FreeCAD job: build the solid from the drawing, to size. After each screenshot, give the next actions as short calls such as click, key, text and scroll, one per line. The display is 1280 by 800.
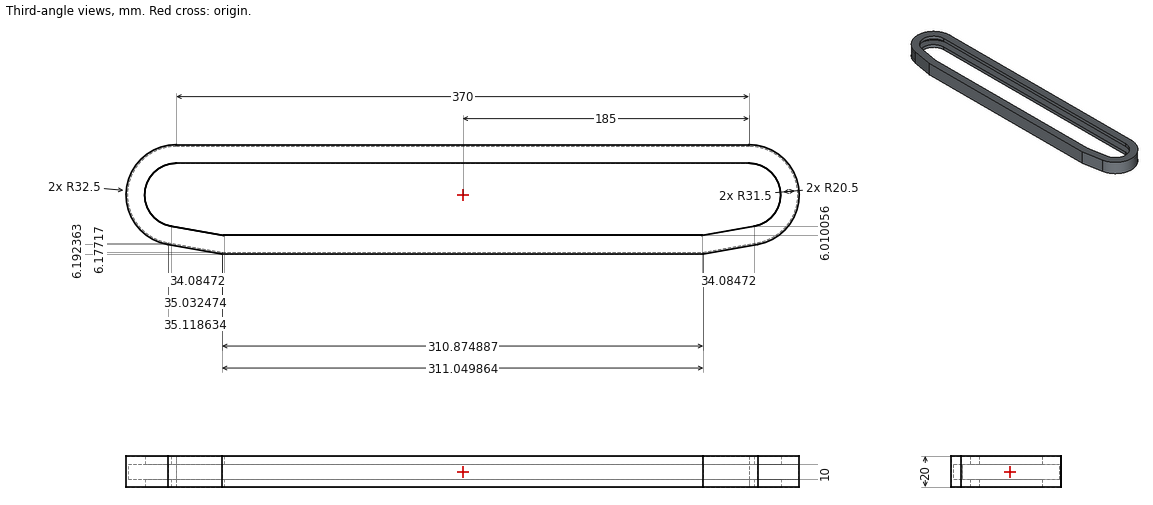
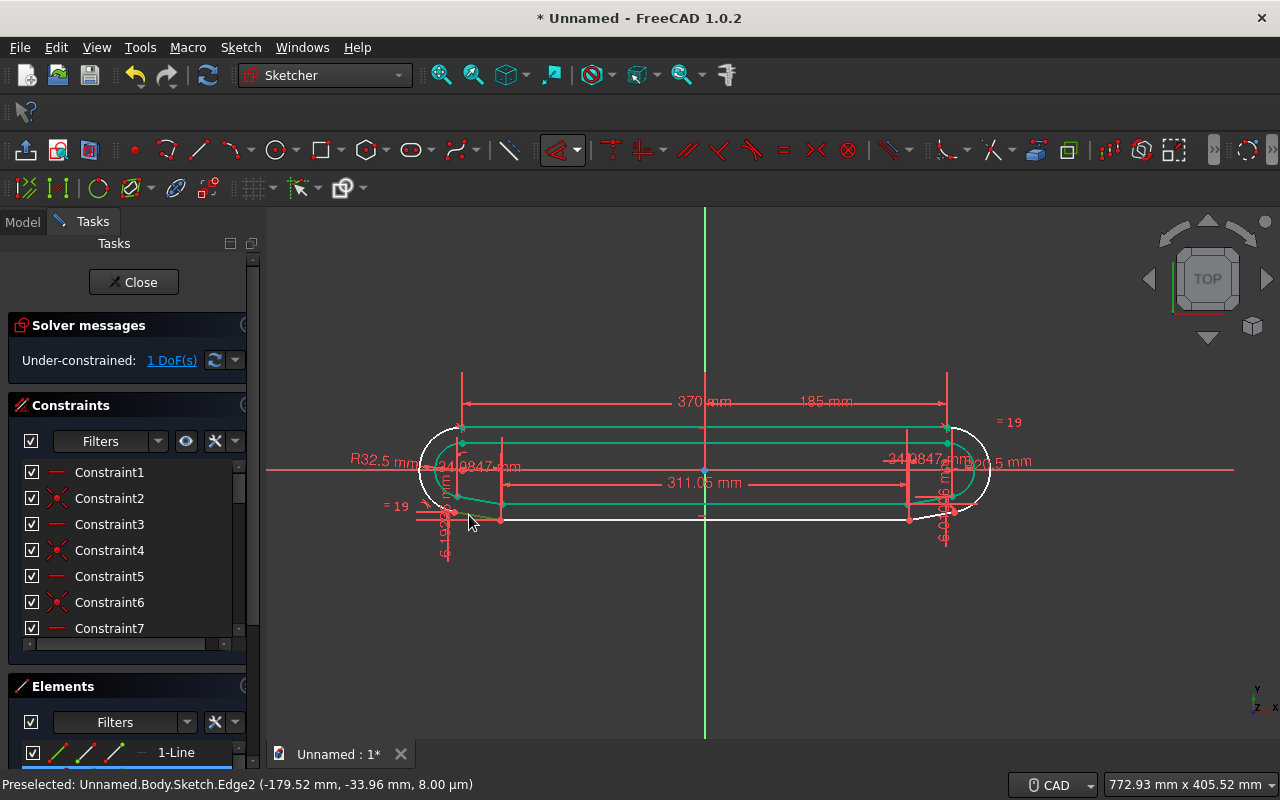
key(l)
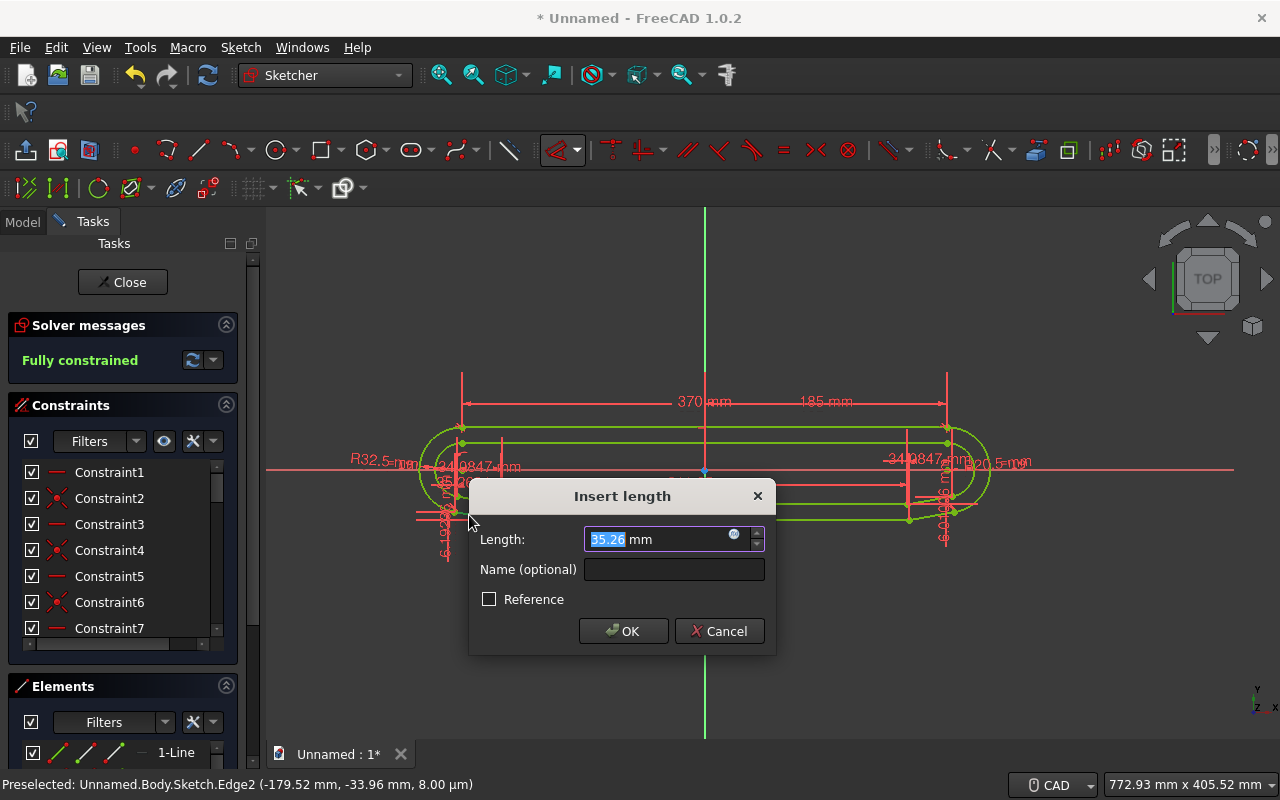
text(35.118634)
key(Return)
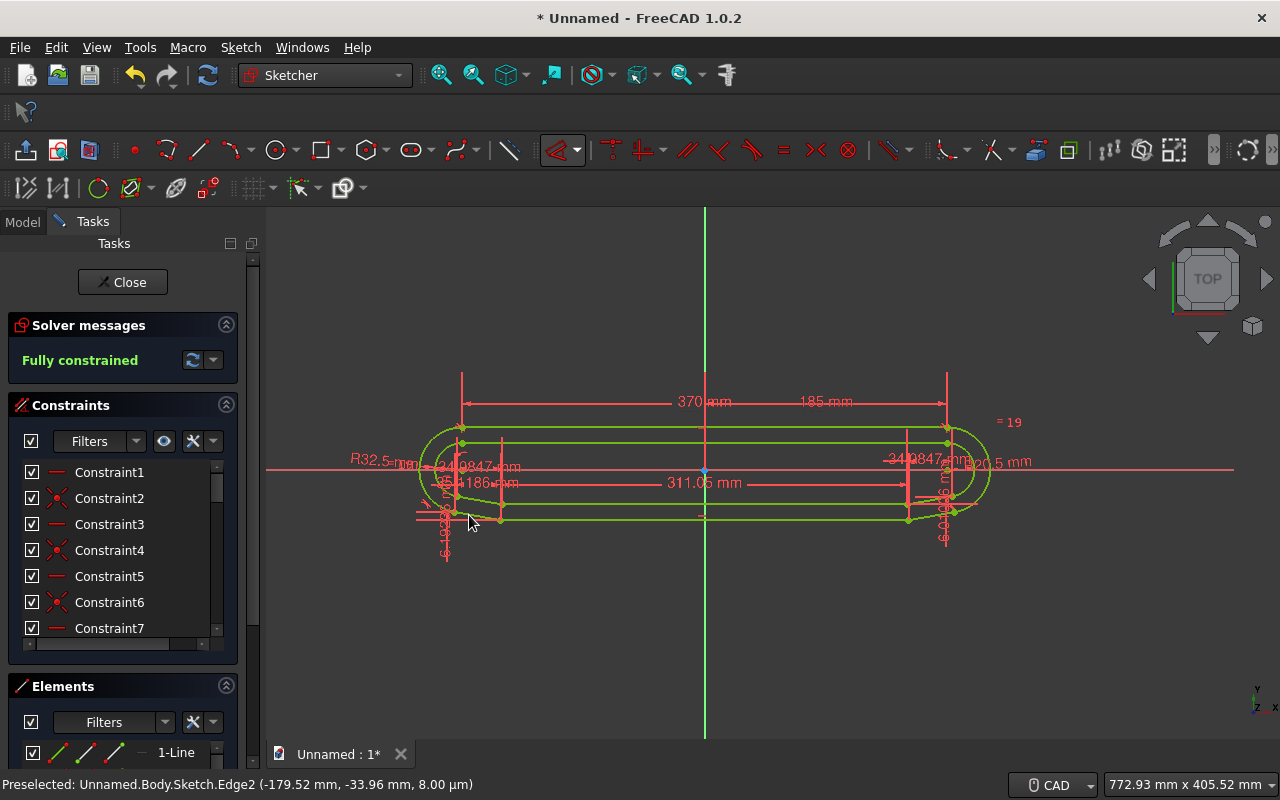
click(123, 282)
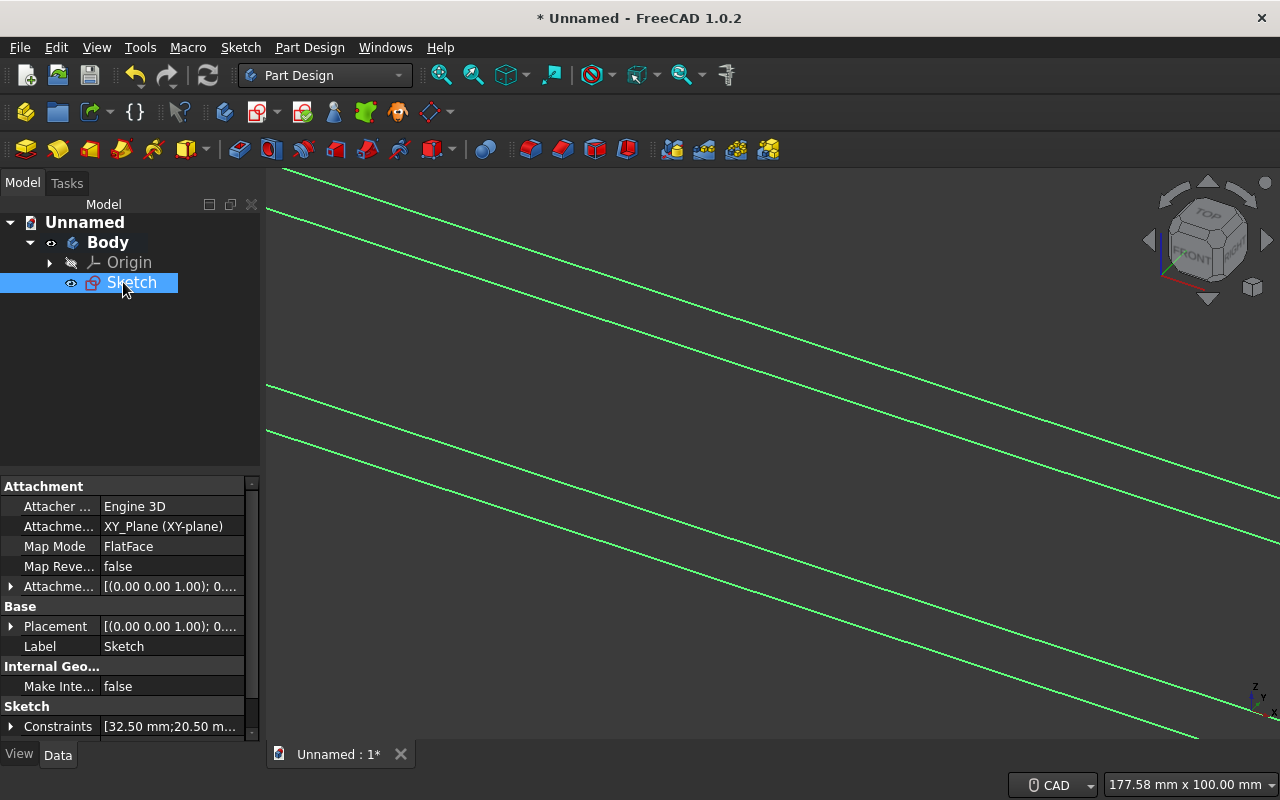
click(26, 150)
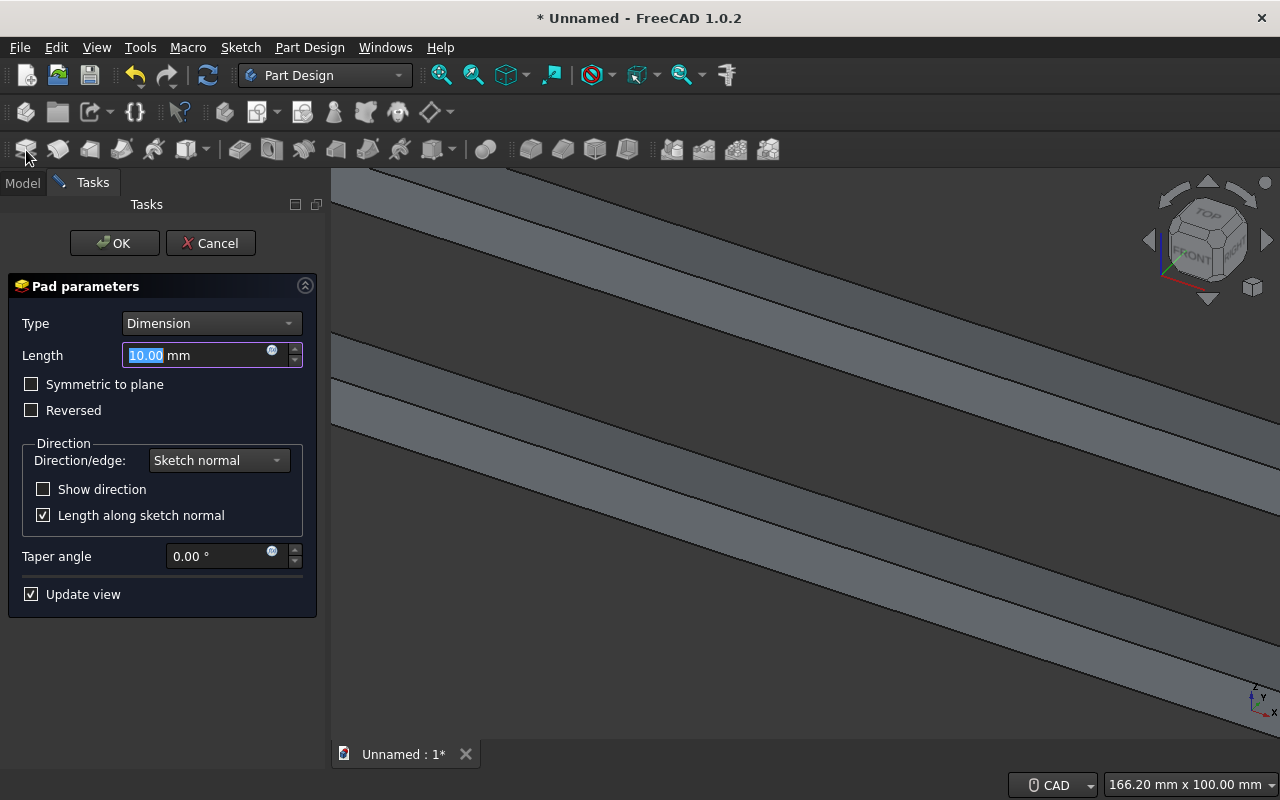
text(20)
key(Tab)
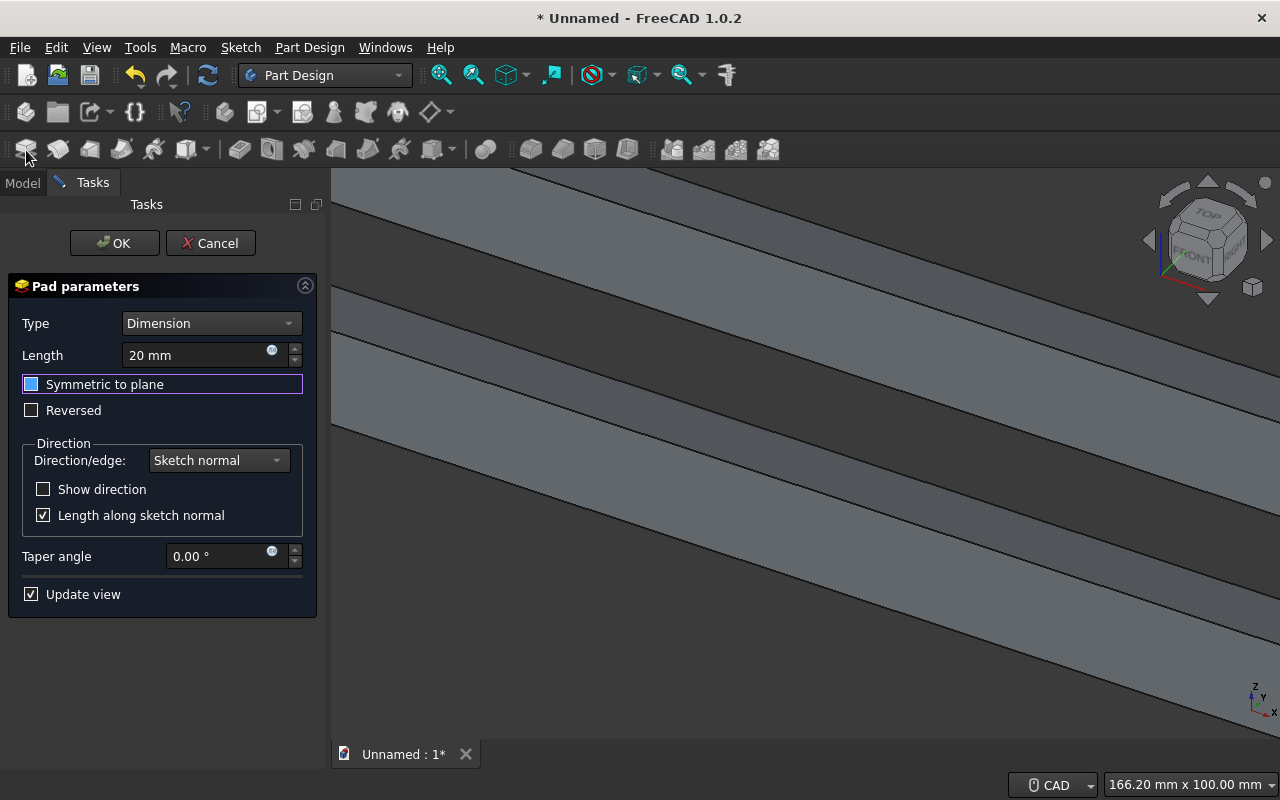
click(30, 384)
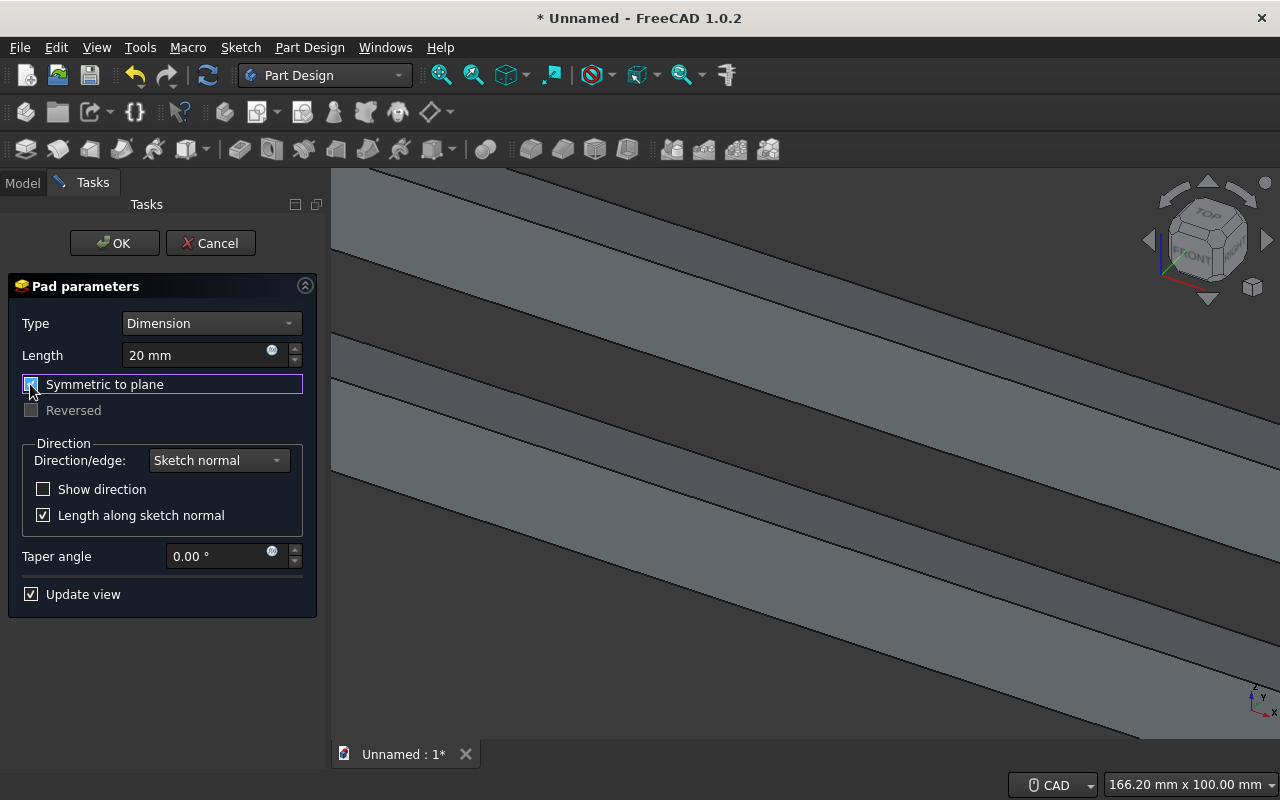
click(115, 243)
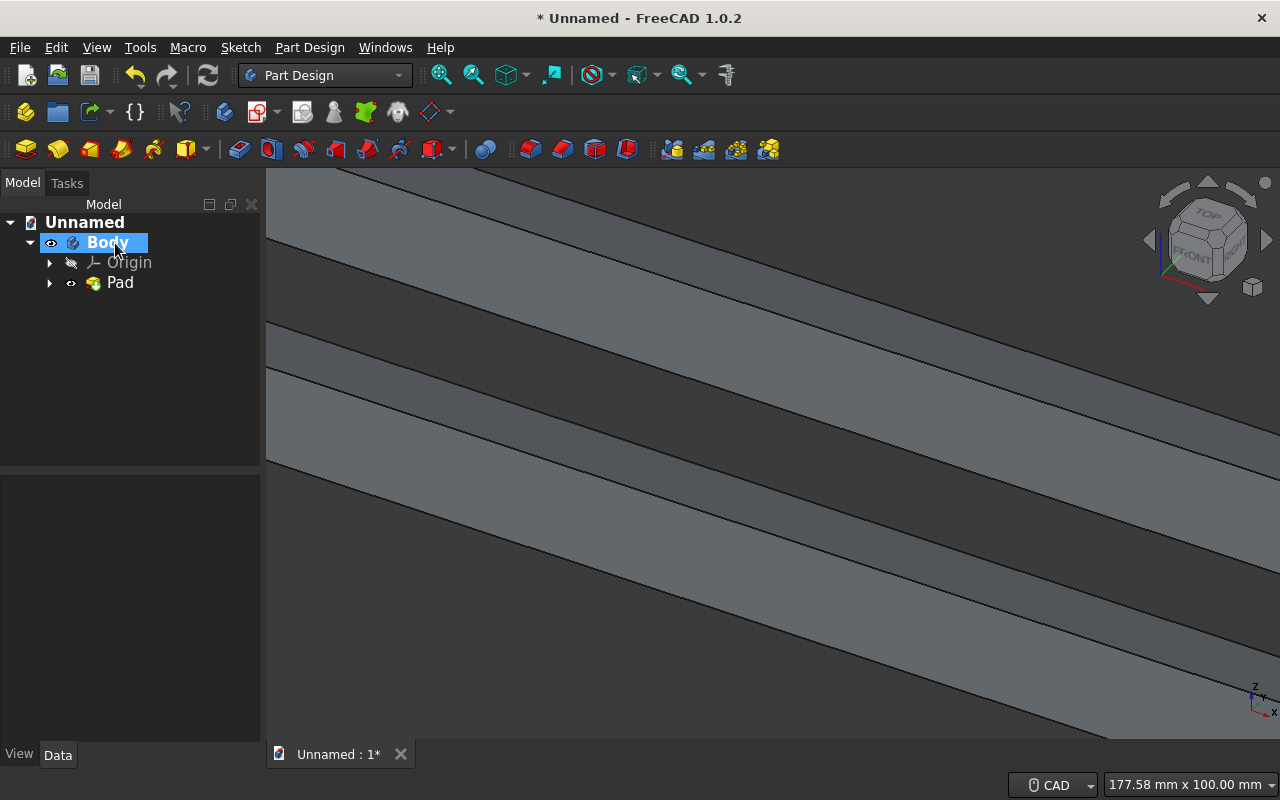
key(v)
key(f)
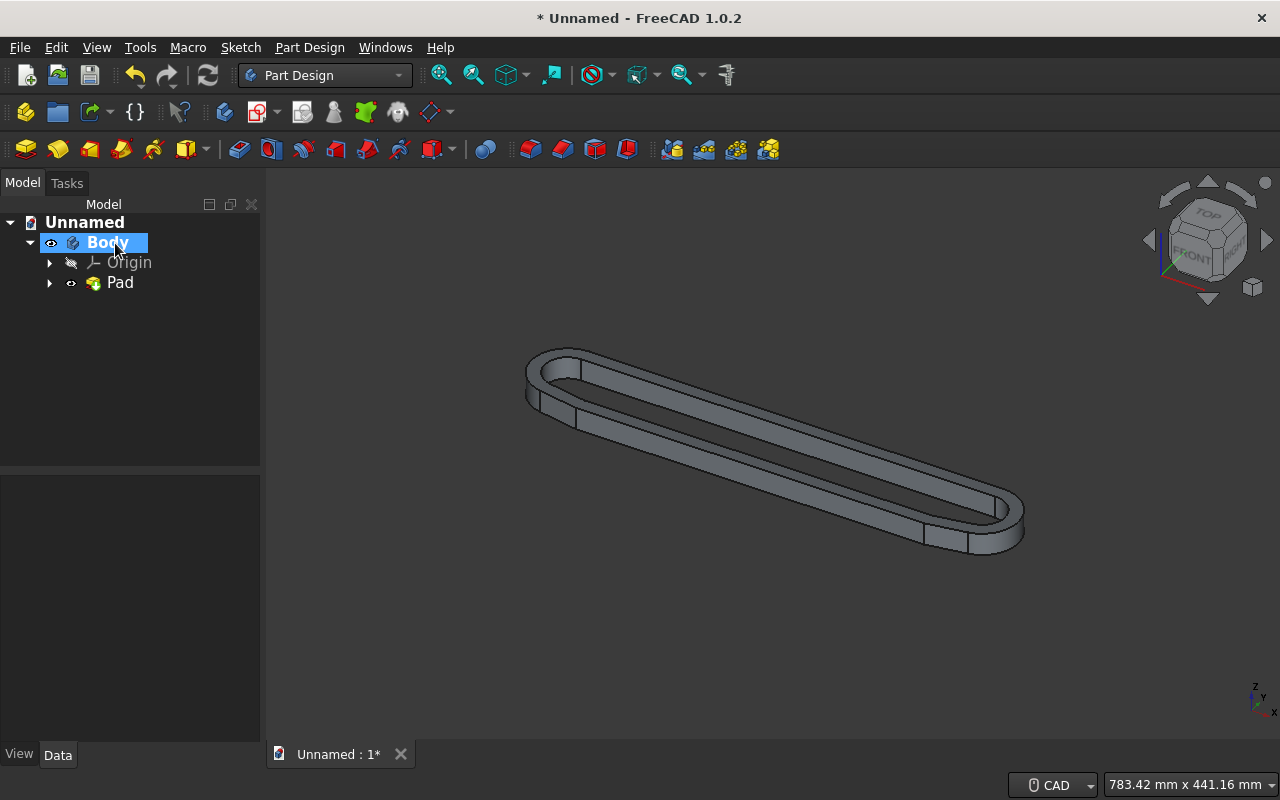
click(258, 112)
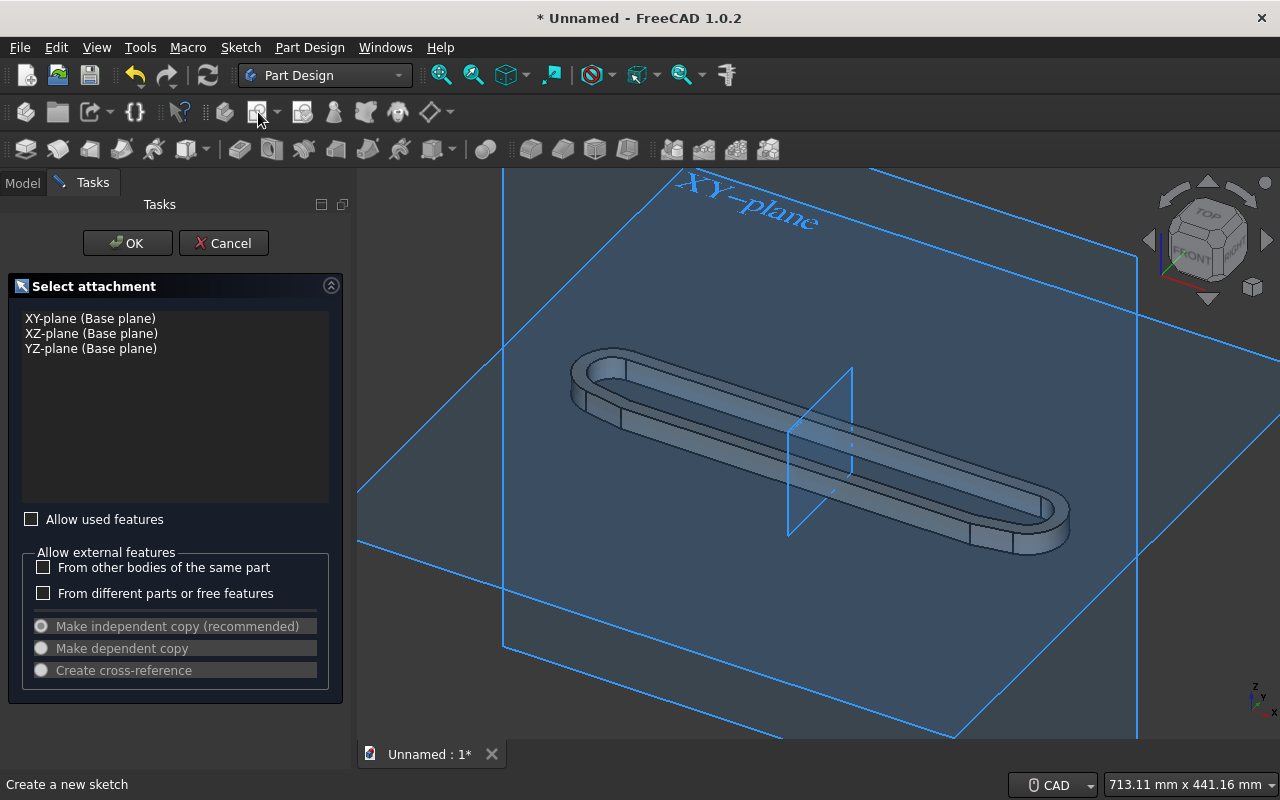
click(82, 318)